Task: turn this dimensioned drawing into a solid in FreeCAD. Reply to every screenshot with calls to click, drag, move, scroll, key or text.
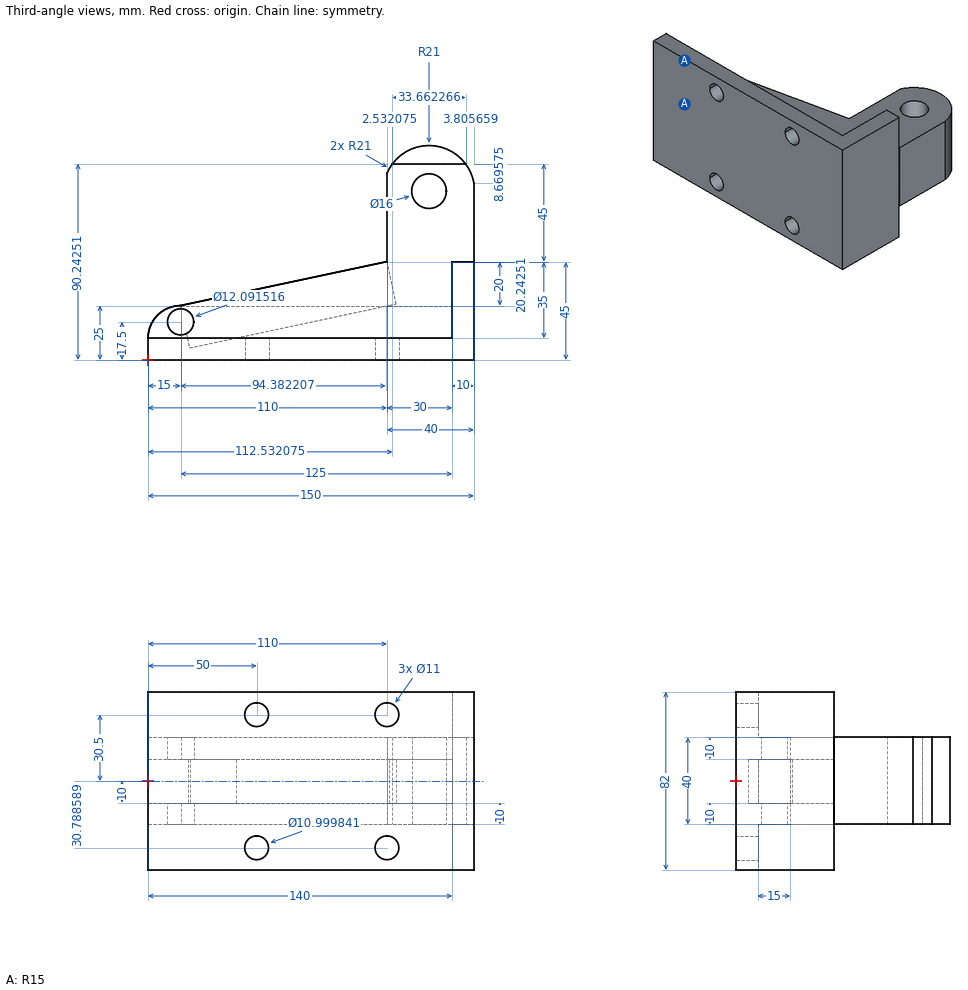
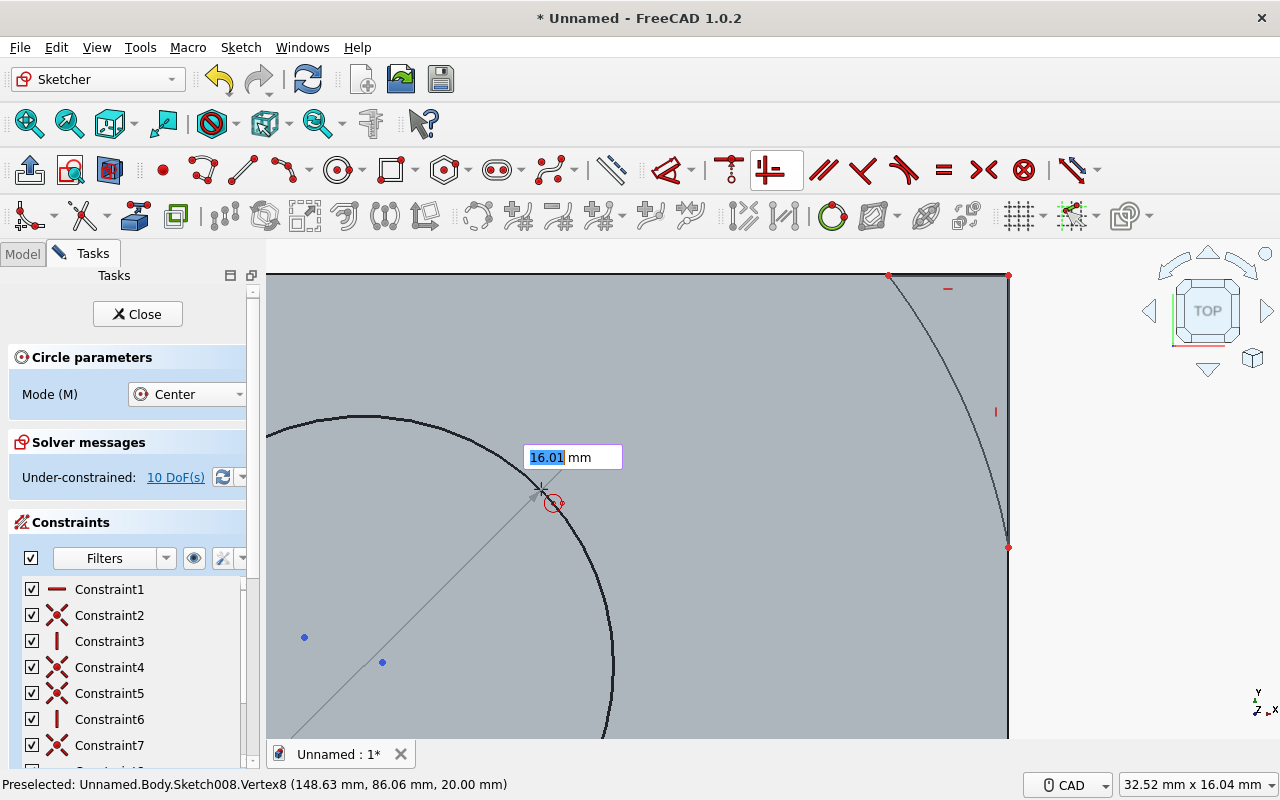
text(16)
key(Return)
key(Escape)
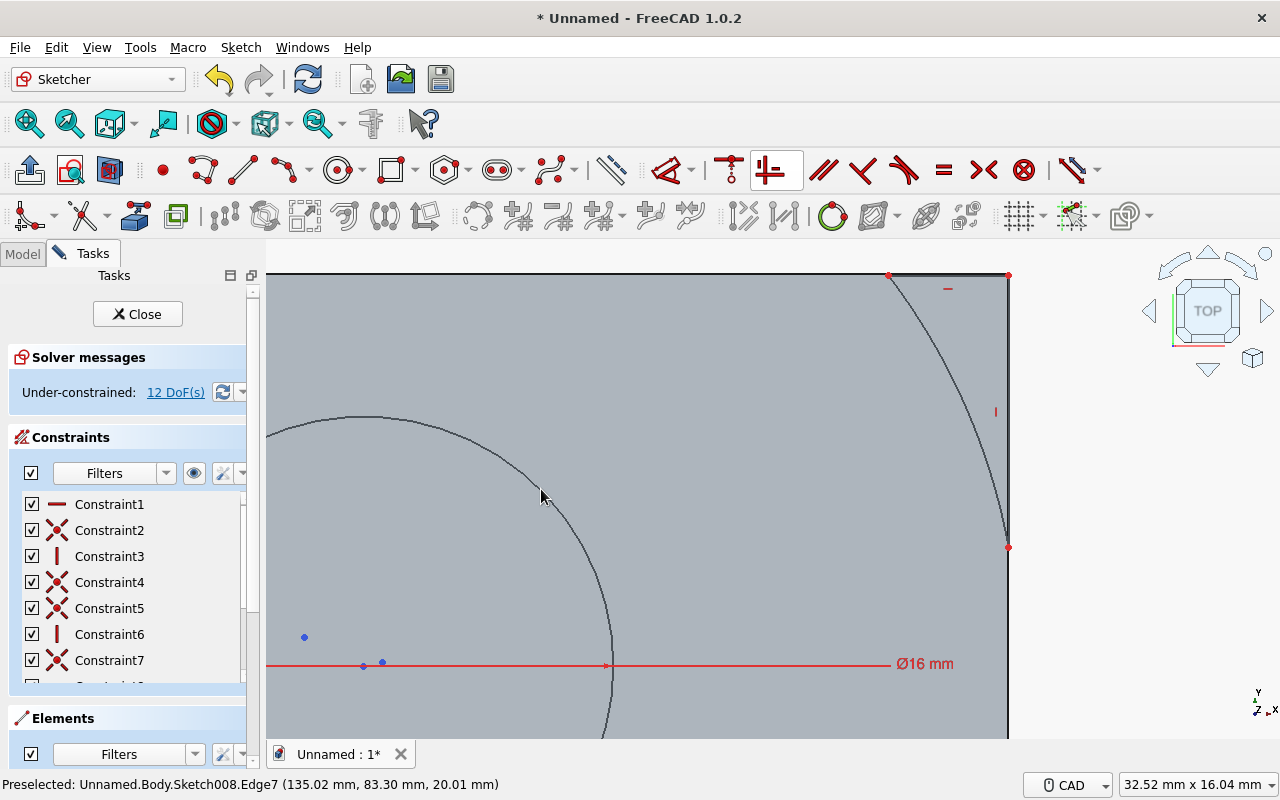
click(540, 489)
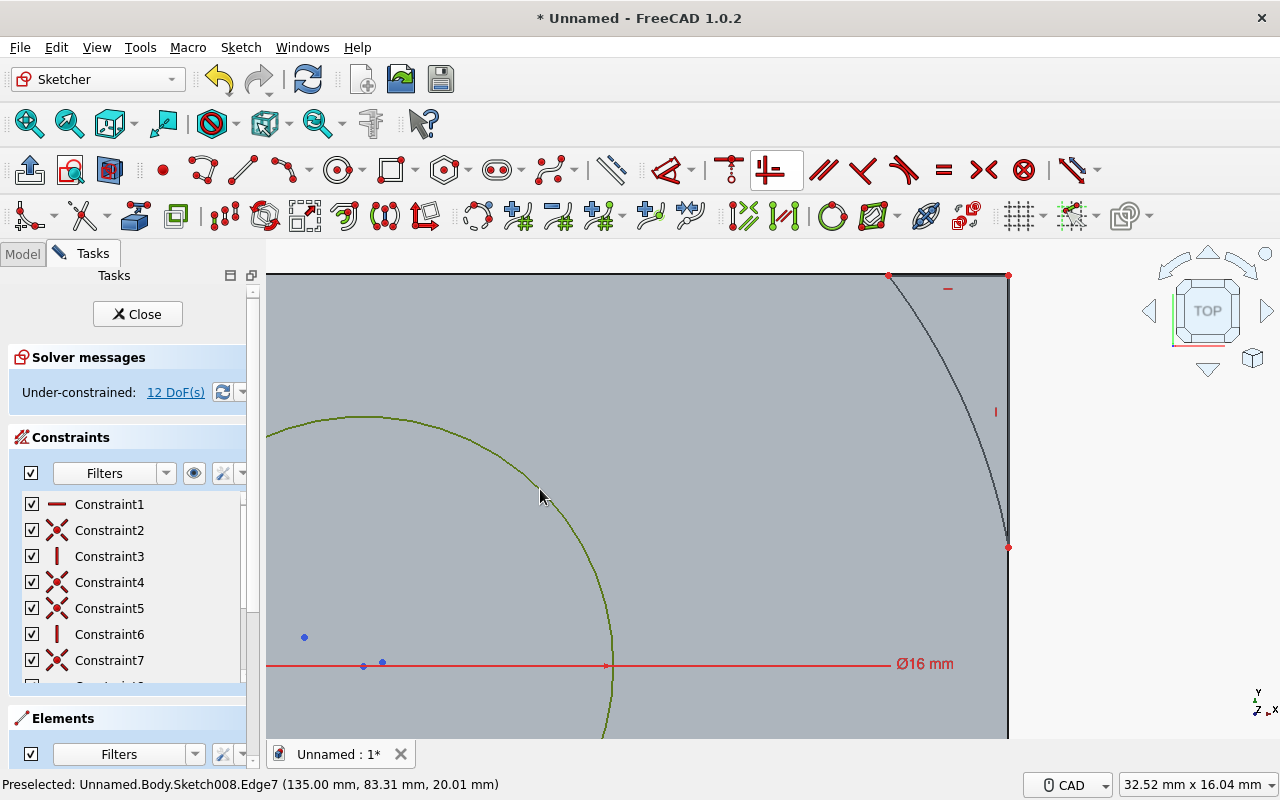
scroll(966, 403, down, 4)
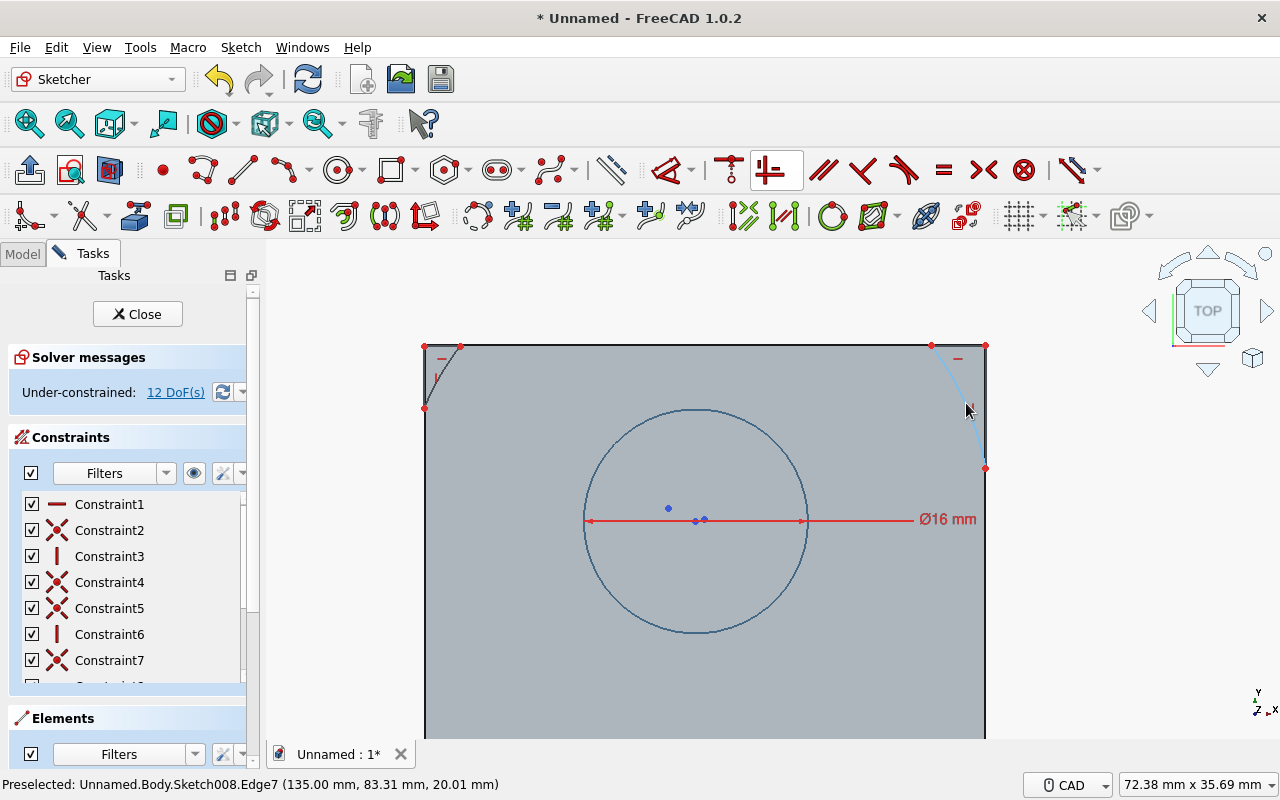
click(448, 364)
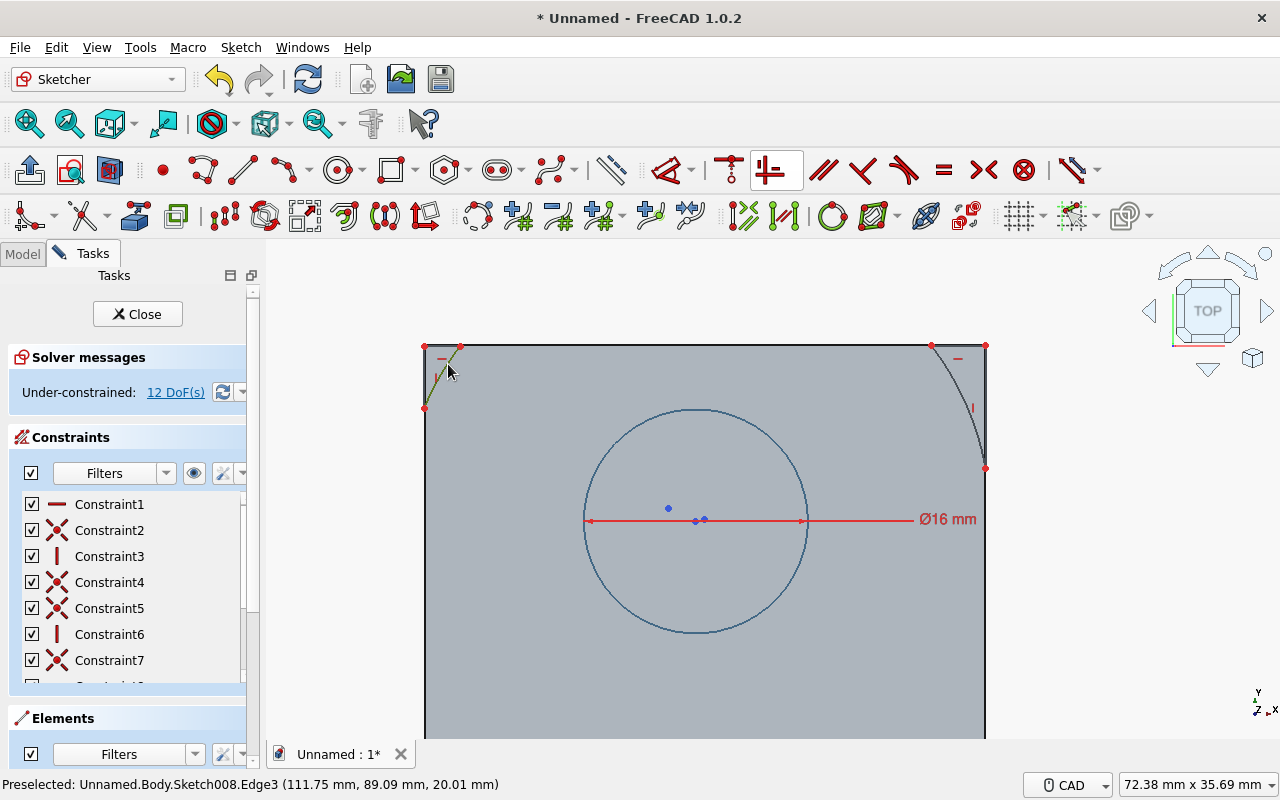
key(c)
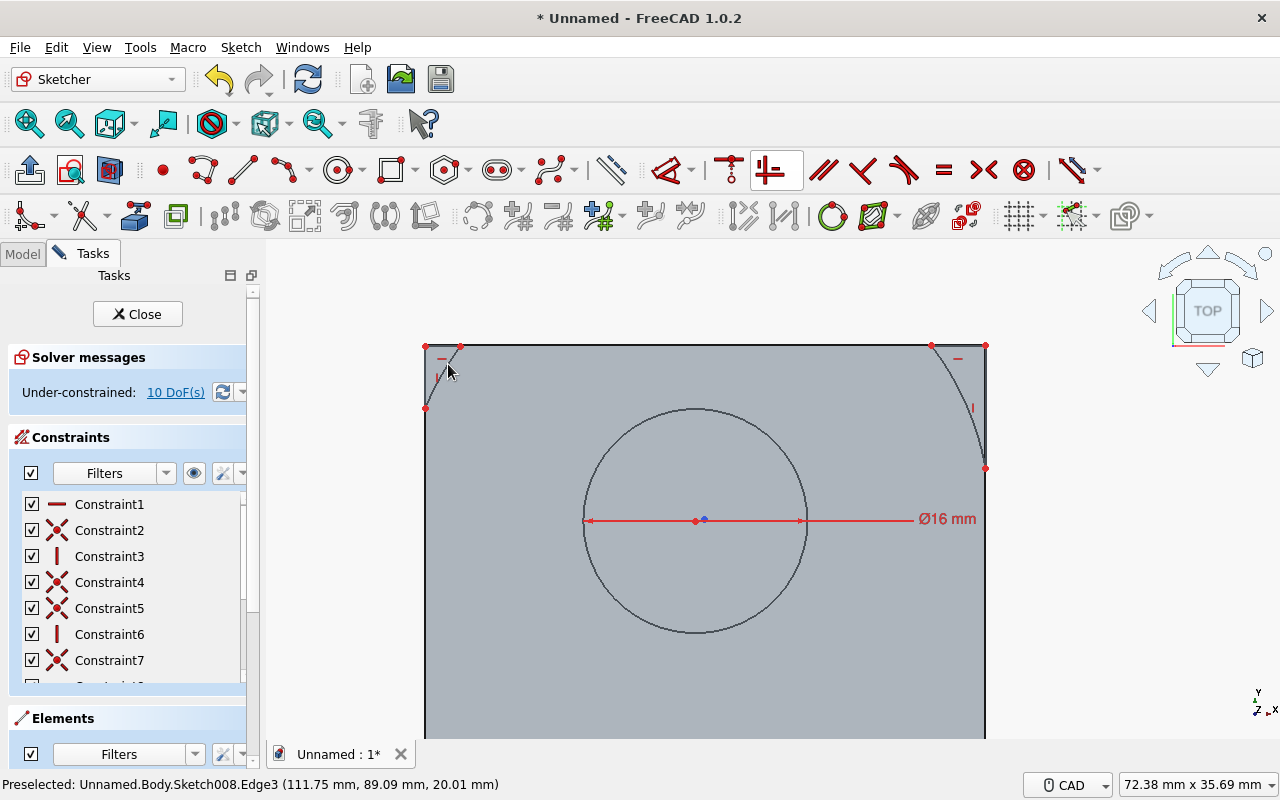
click(774, 442)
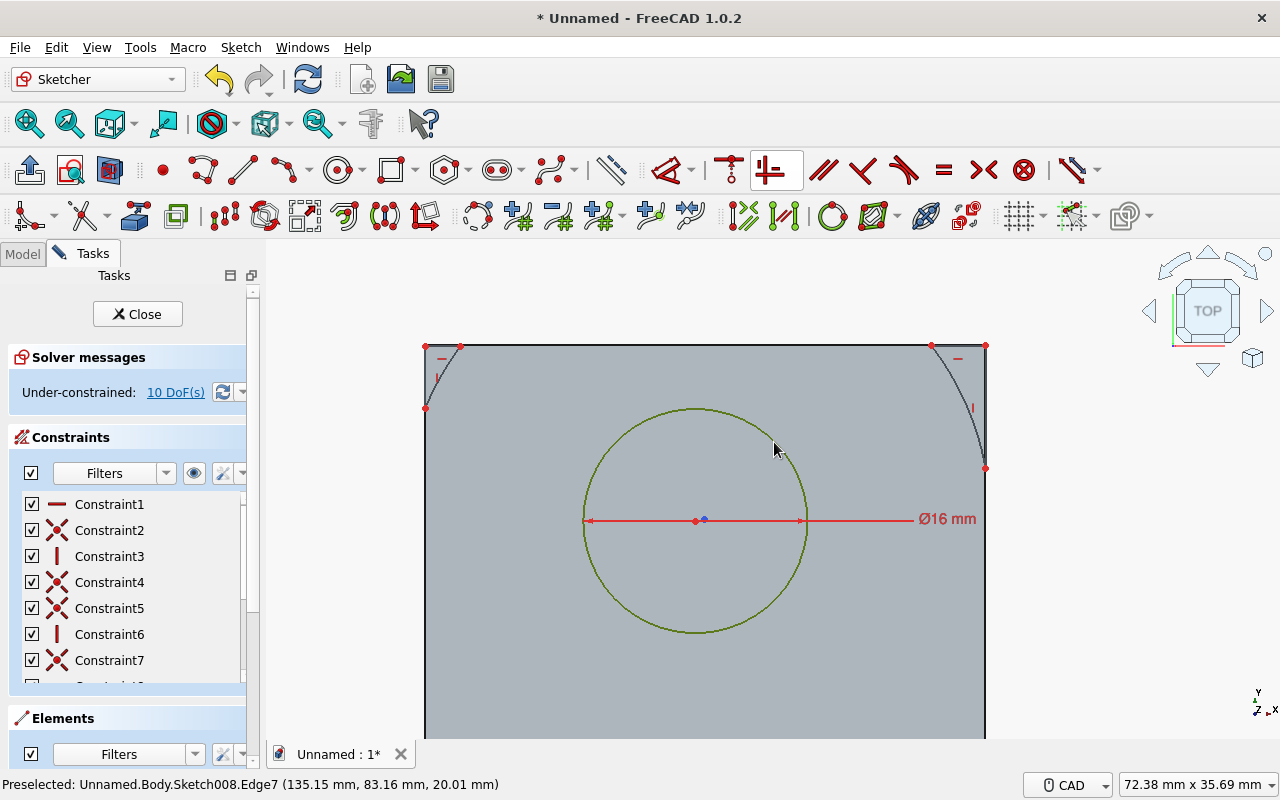
scroll(975, 429, up, 2)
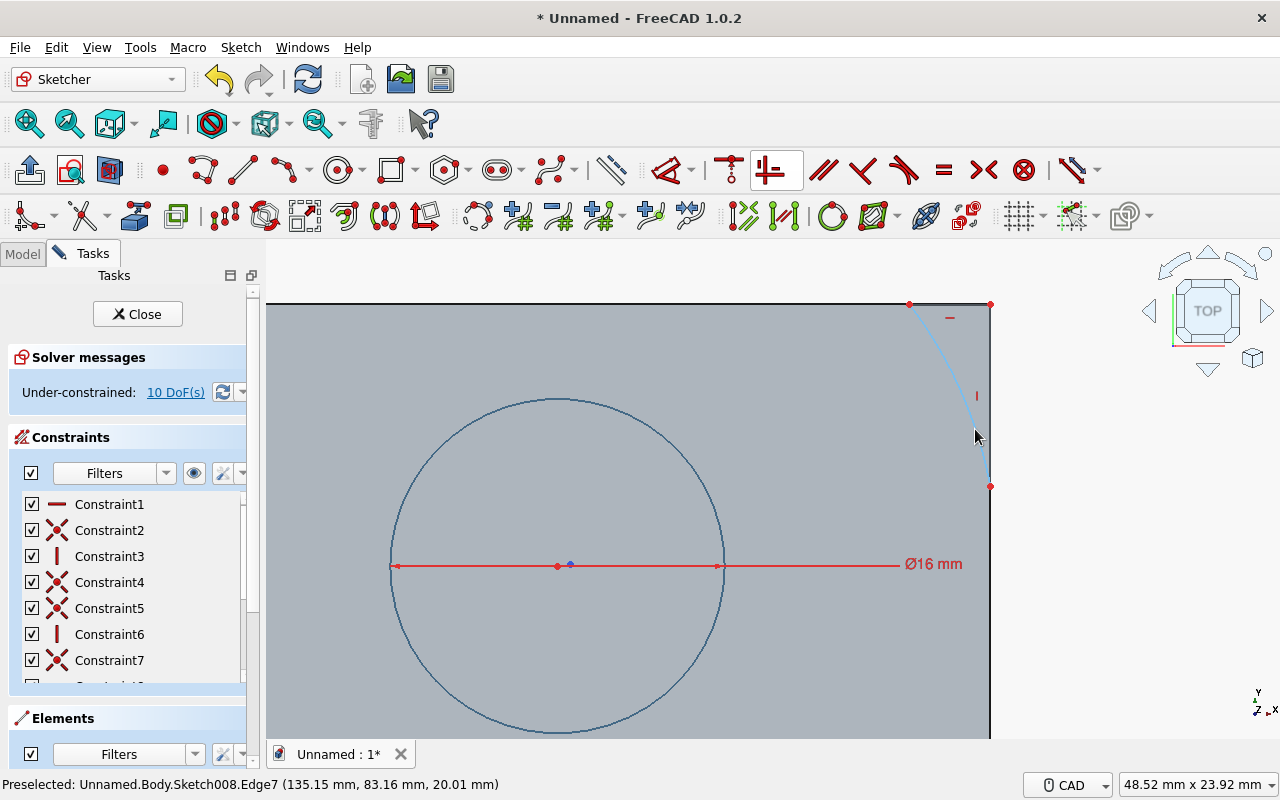
click(975, 429)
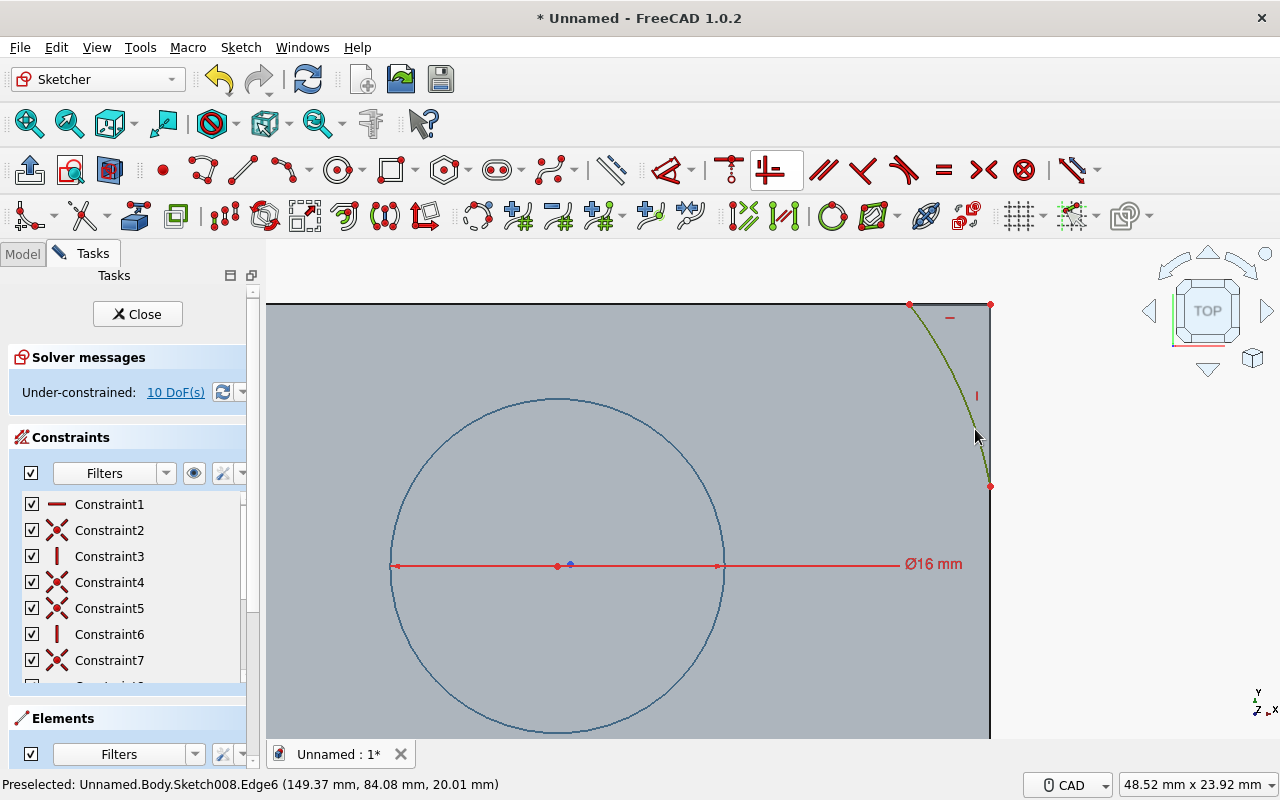
click(730, 170)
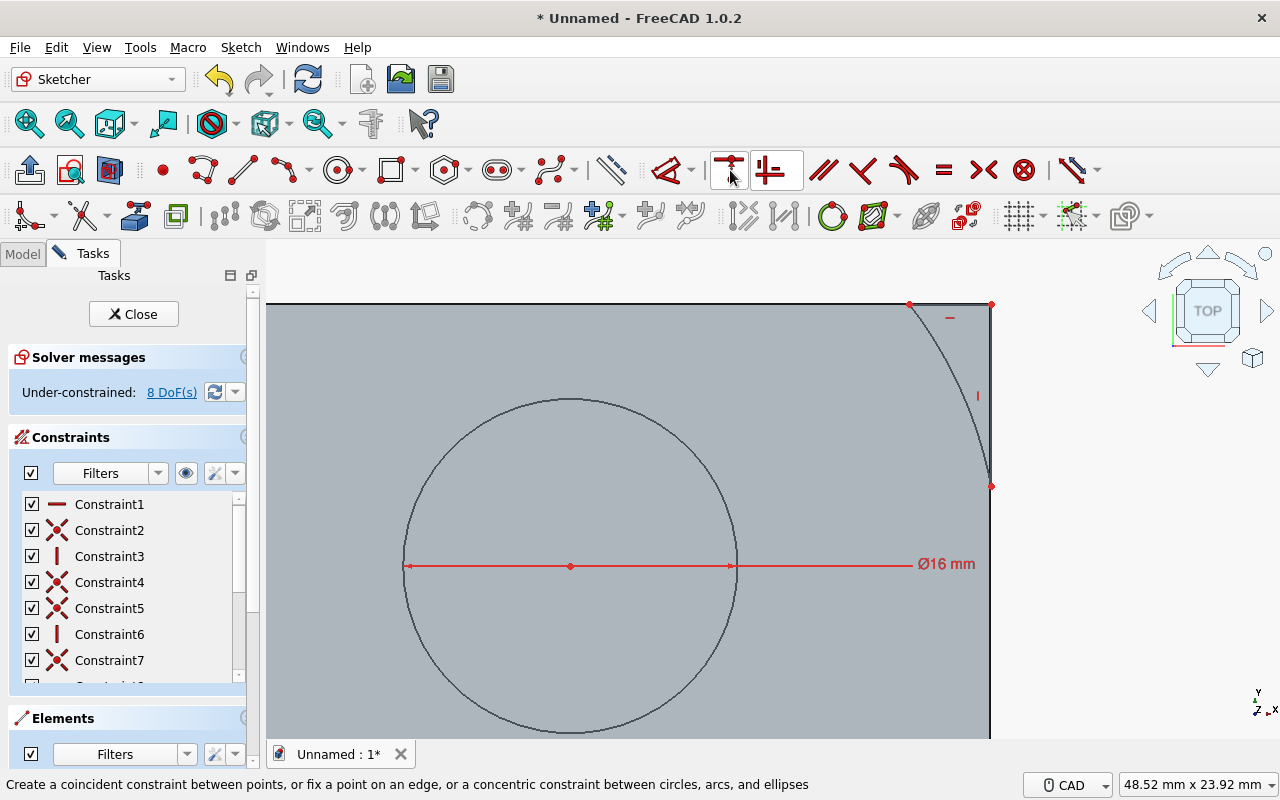
scroll(974, 429, down, 2)